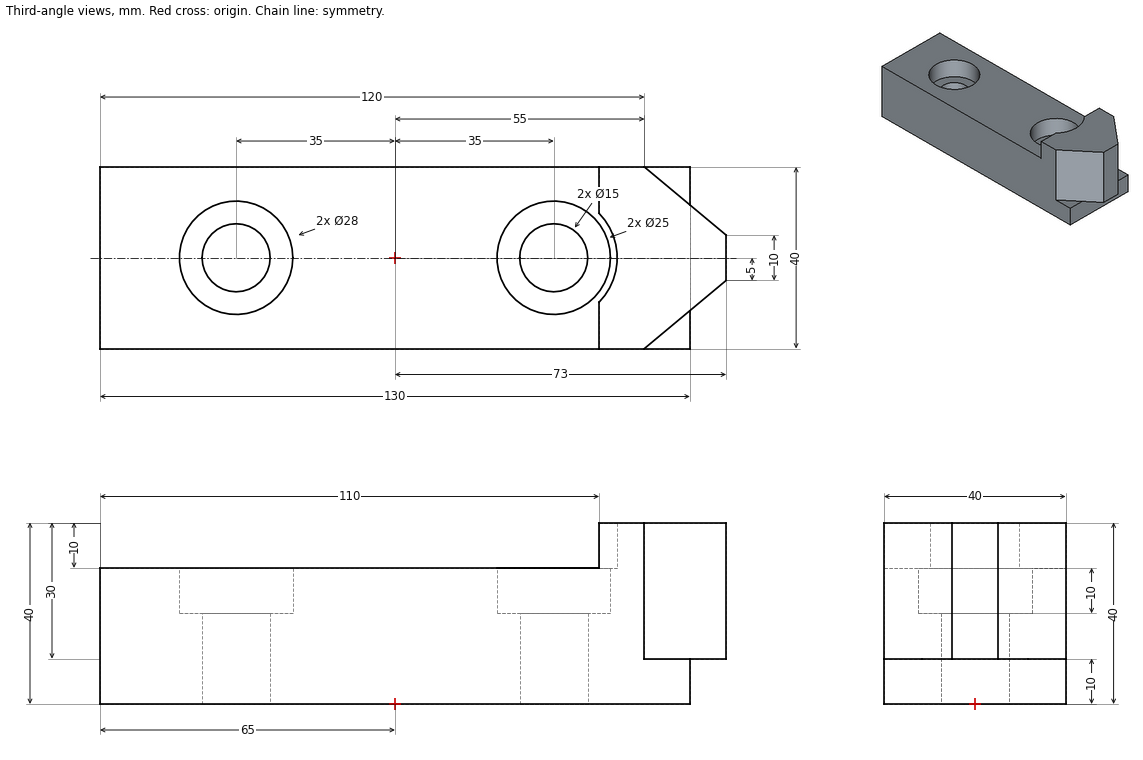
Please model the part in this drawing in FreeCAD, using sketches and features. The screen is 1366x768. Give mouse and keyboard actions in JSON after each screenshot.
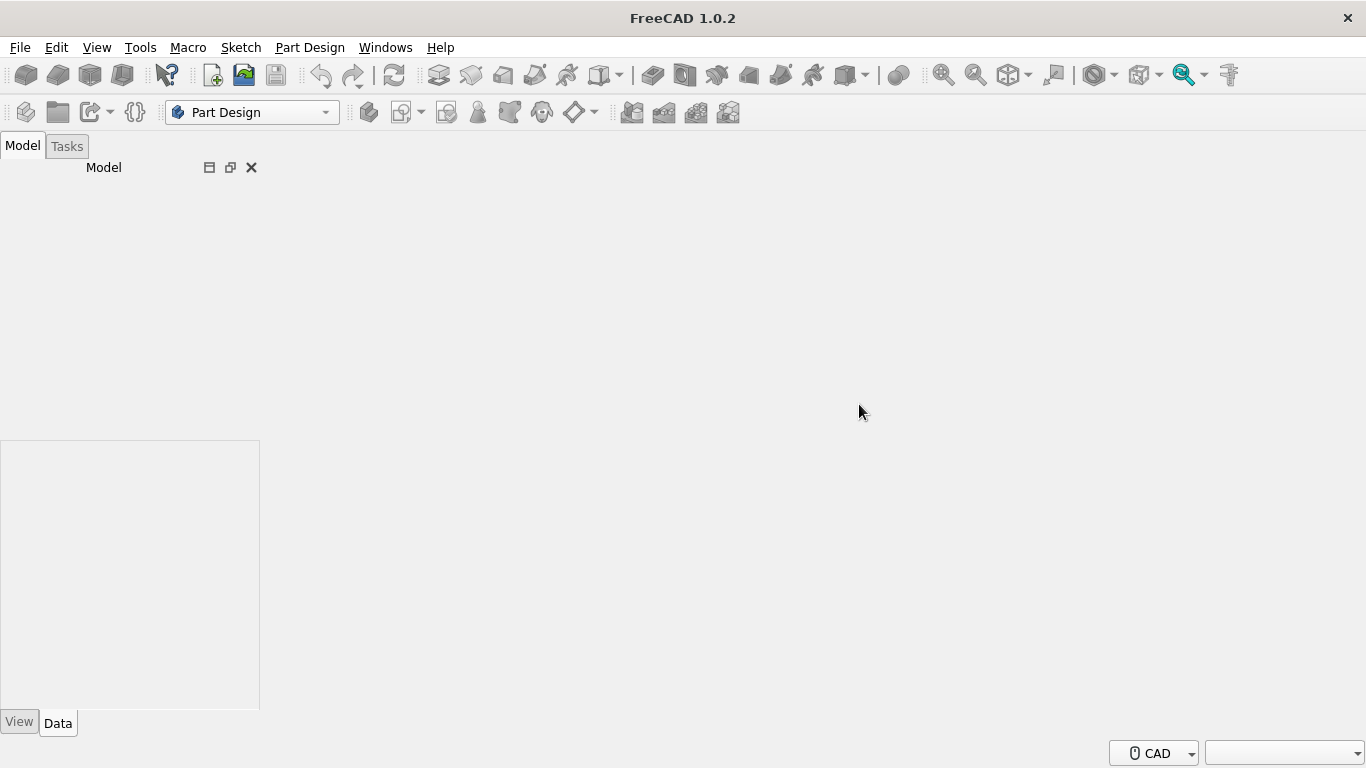
{"action": "left_click", "coordinate": [212, 76]}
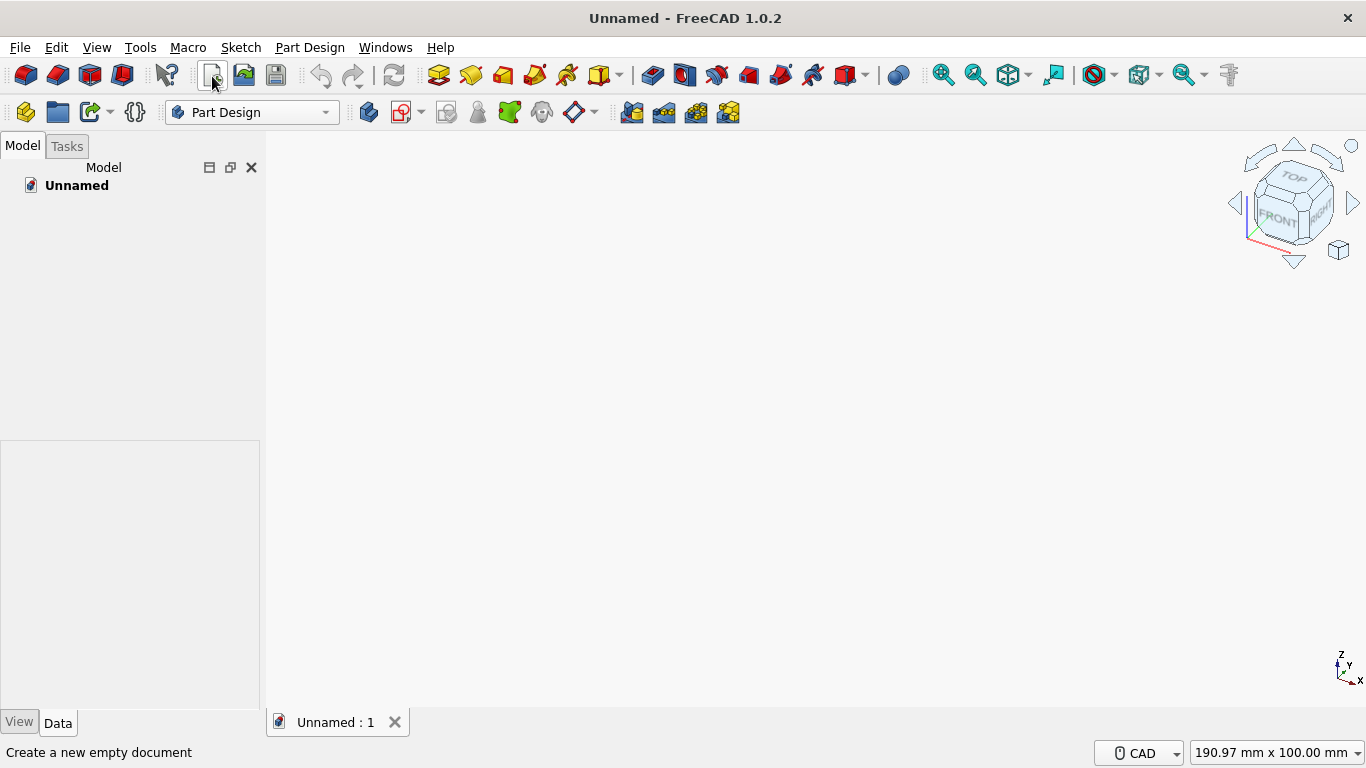
{"action": "left_click", "coordinate": [402, 112]}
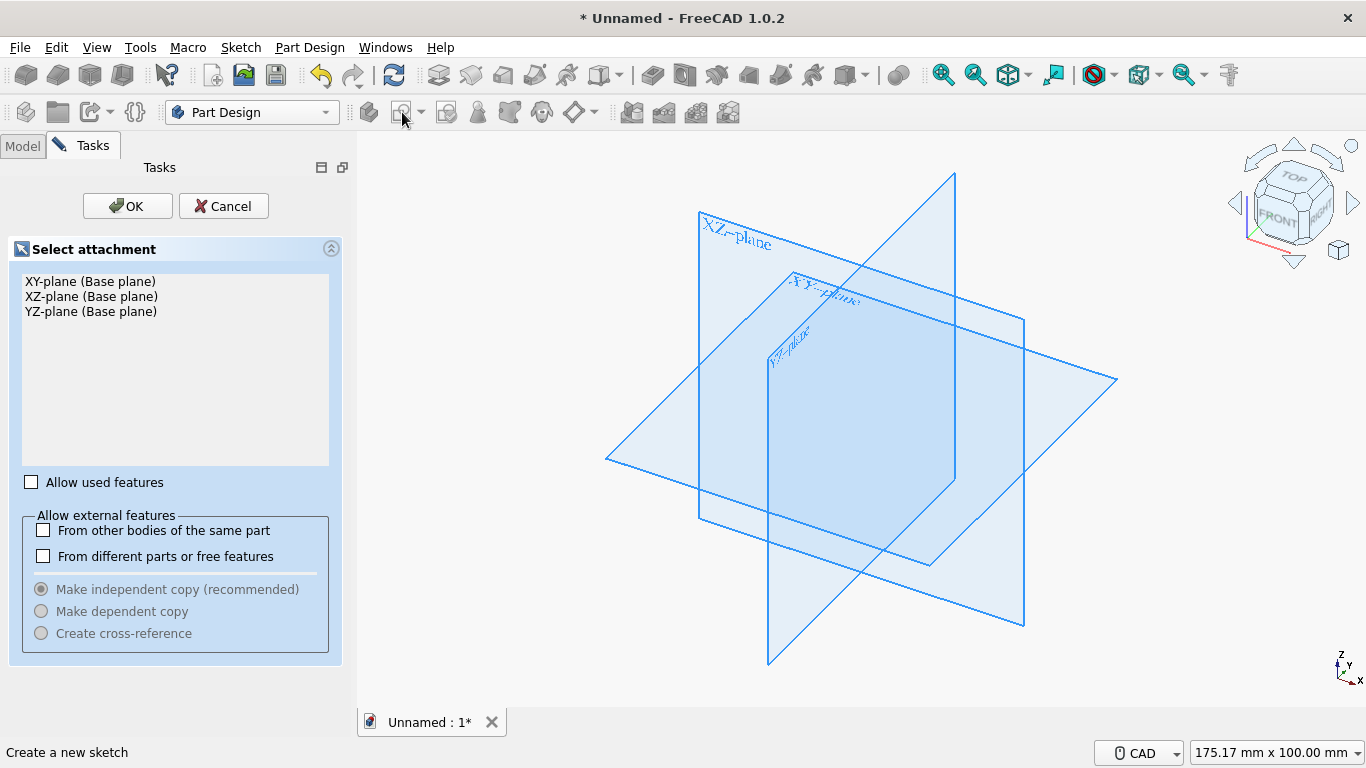
{"action": "left_click", "coordinate": [82, 282]}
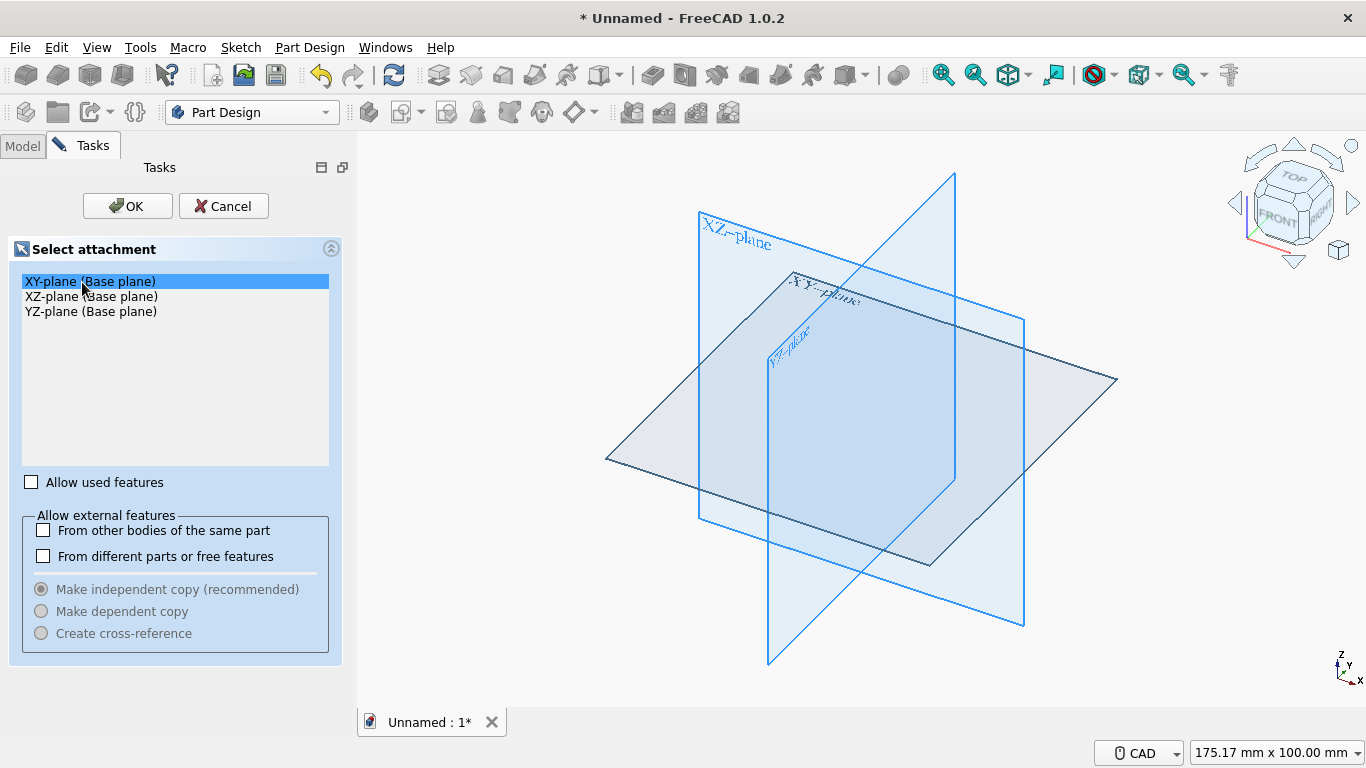
{"action": "left_click", "coordinate": [128, 206]}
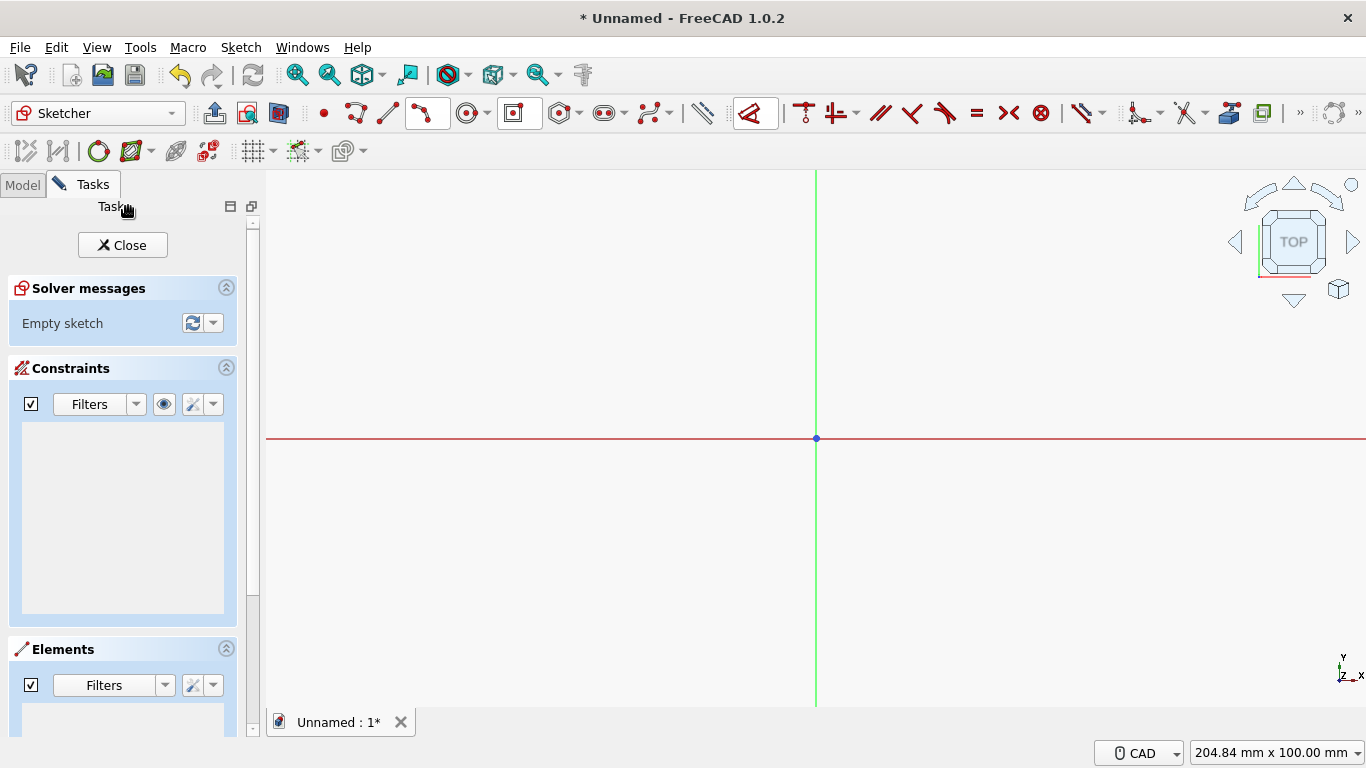
{"action": "left_click", "coordinate": [514, 114]}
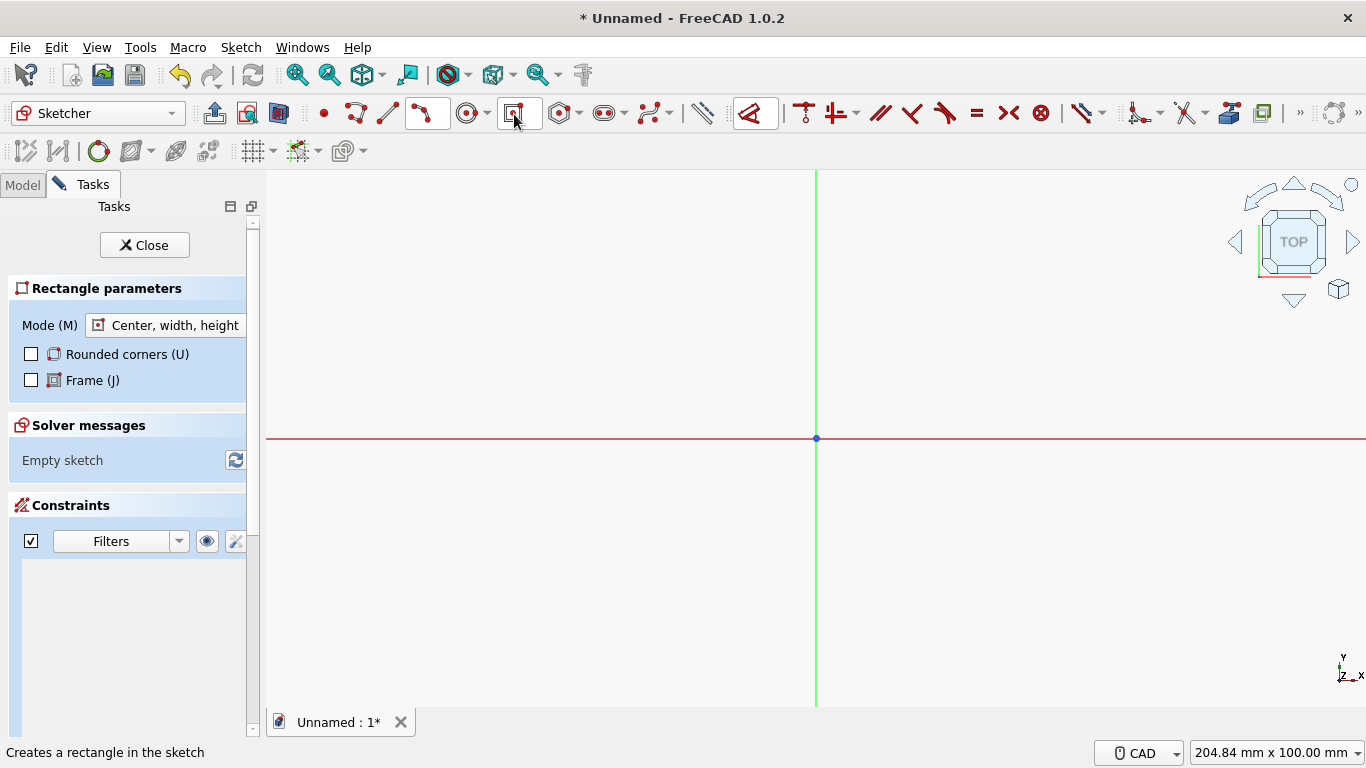
{"action": "left_click", "coordinate": [816, 438]}
{"action": "left_click", "coordinate": [1165, 331]}
{"action": "key", "text": "Escape"}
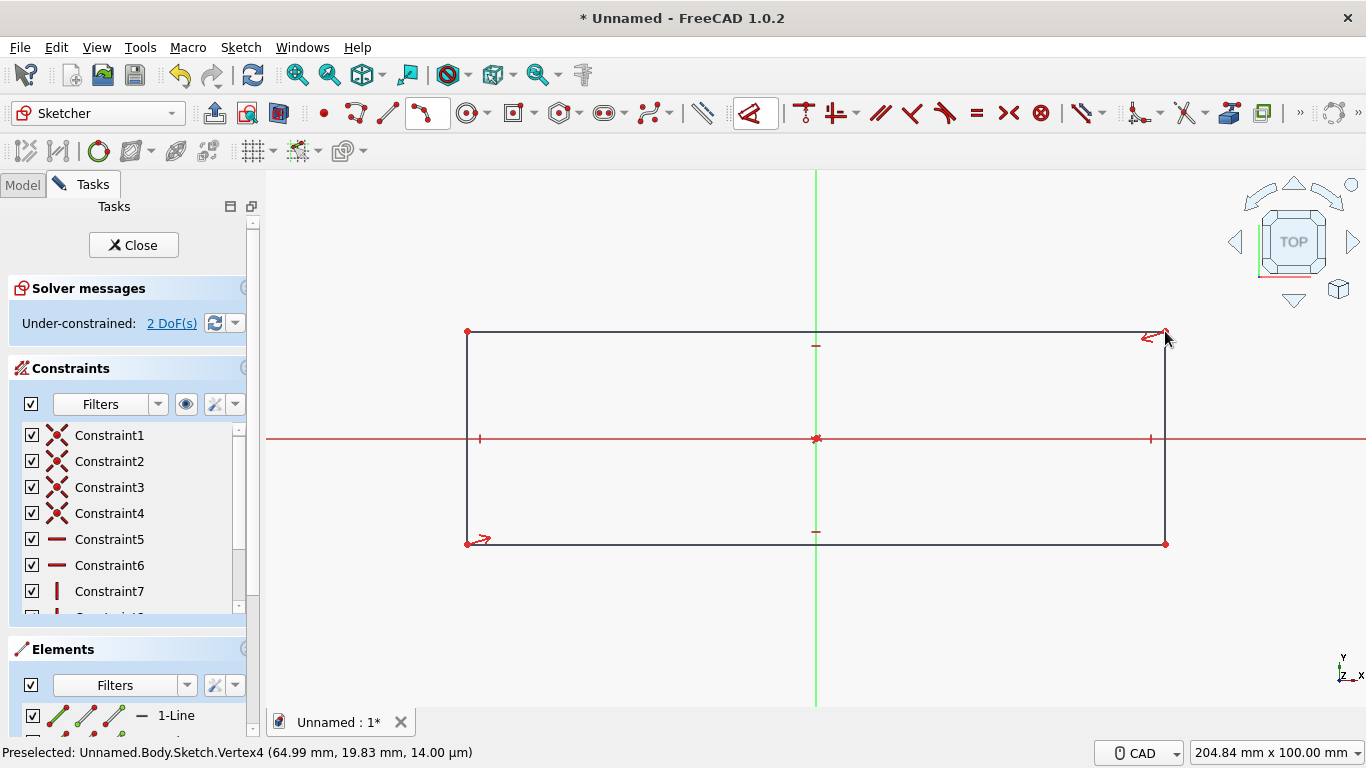
{"action": "left_click", "coordinate": [750, 114]}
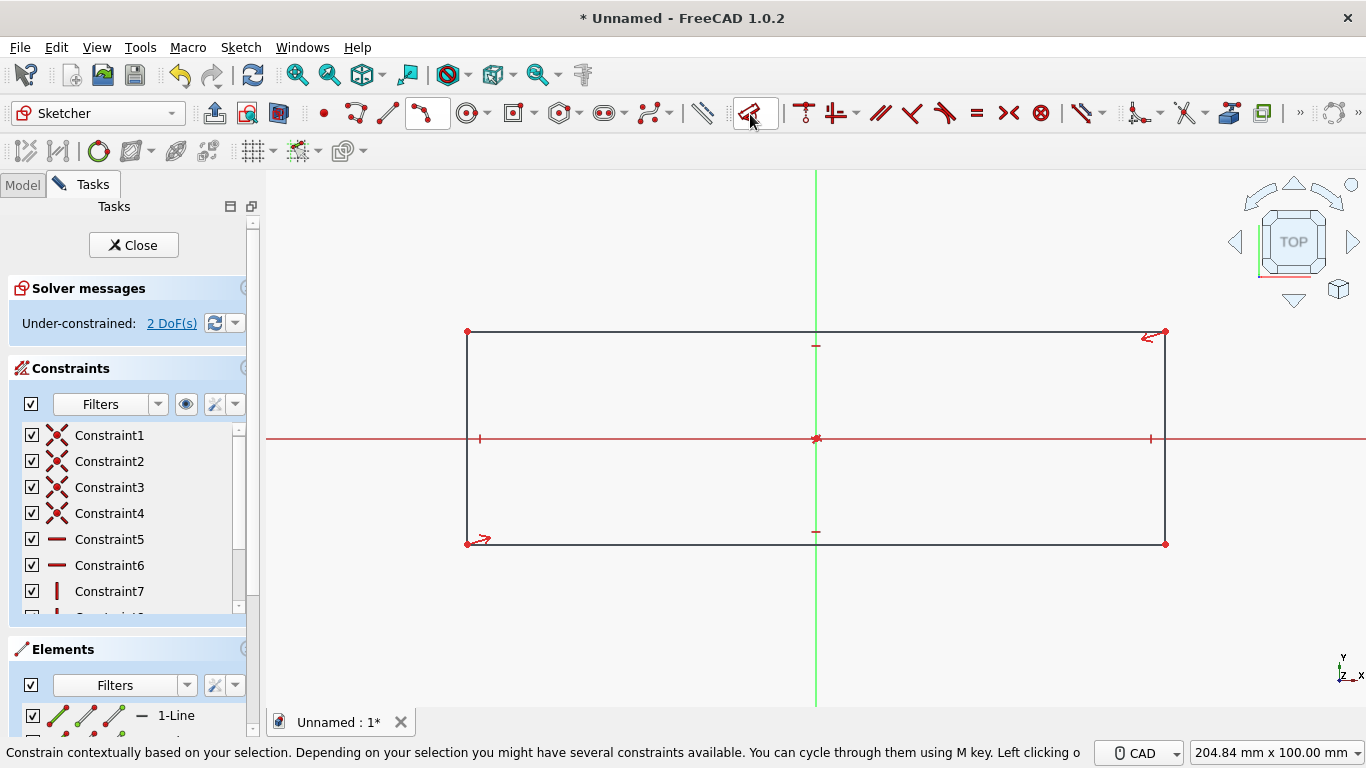
{"action": "left_click", "coordinate": [1165, 481]}
{"action": "left_click", "coordinate": [1199, 390]}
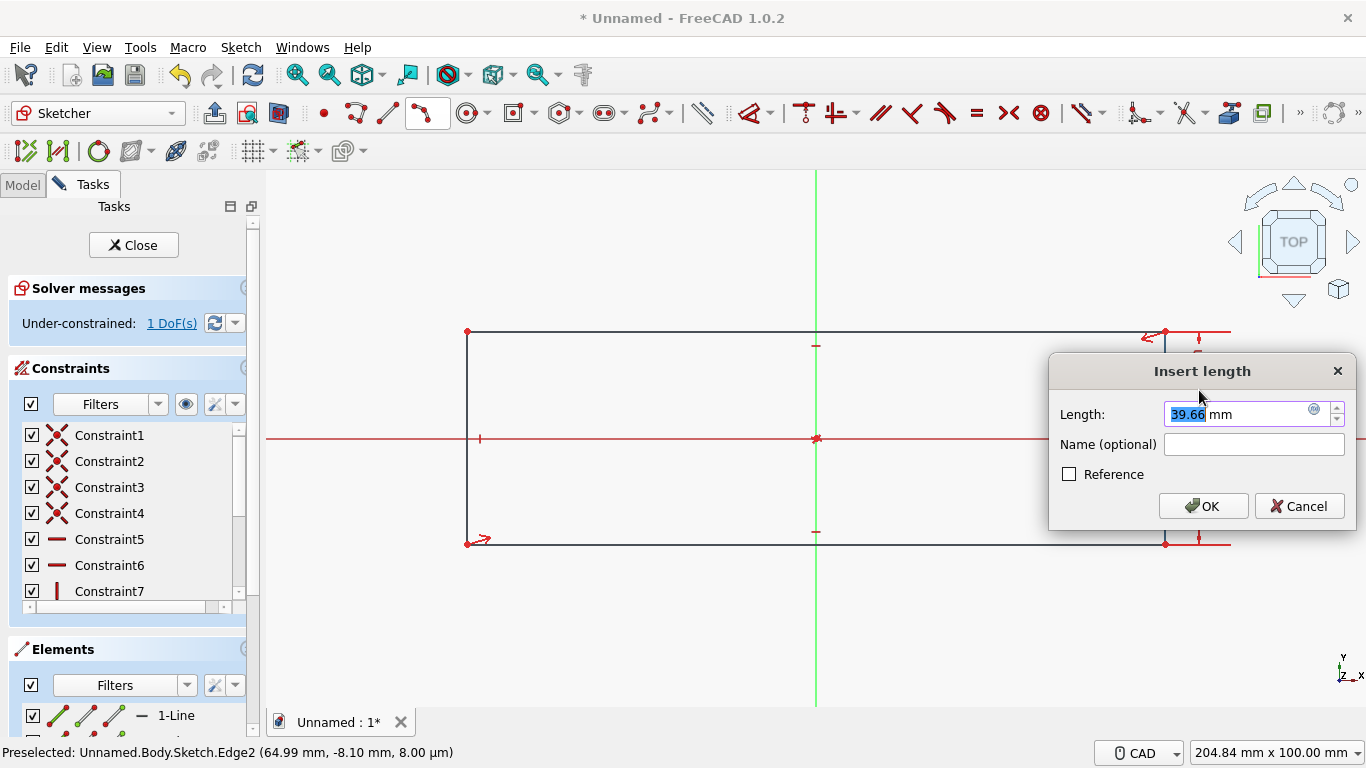
{"action": "type", "text": "40"}
{"action": "key", "text": "Return"}